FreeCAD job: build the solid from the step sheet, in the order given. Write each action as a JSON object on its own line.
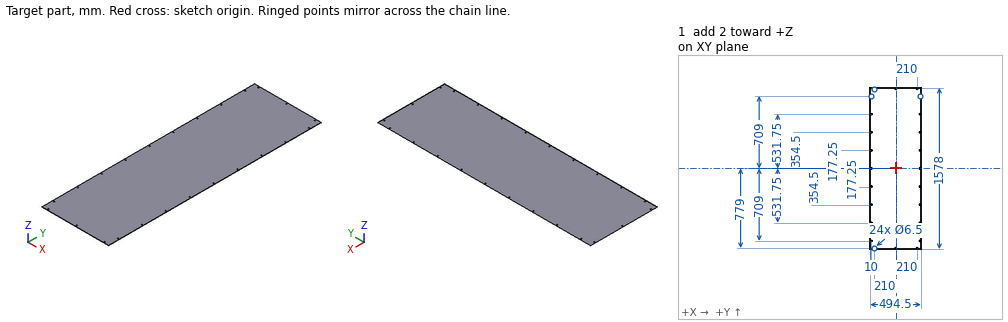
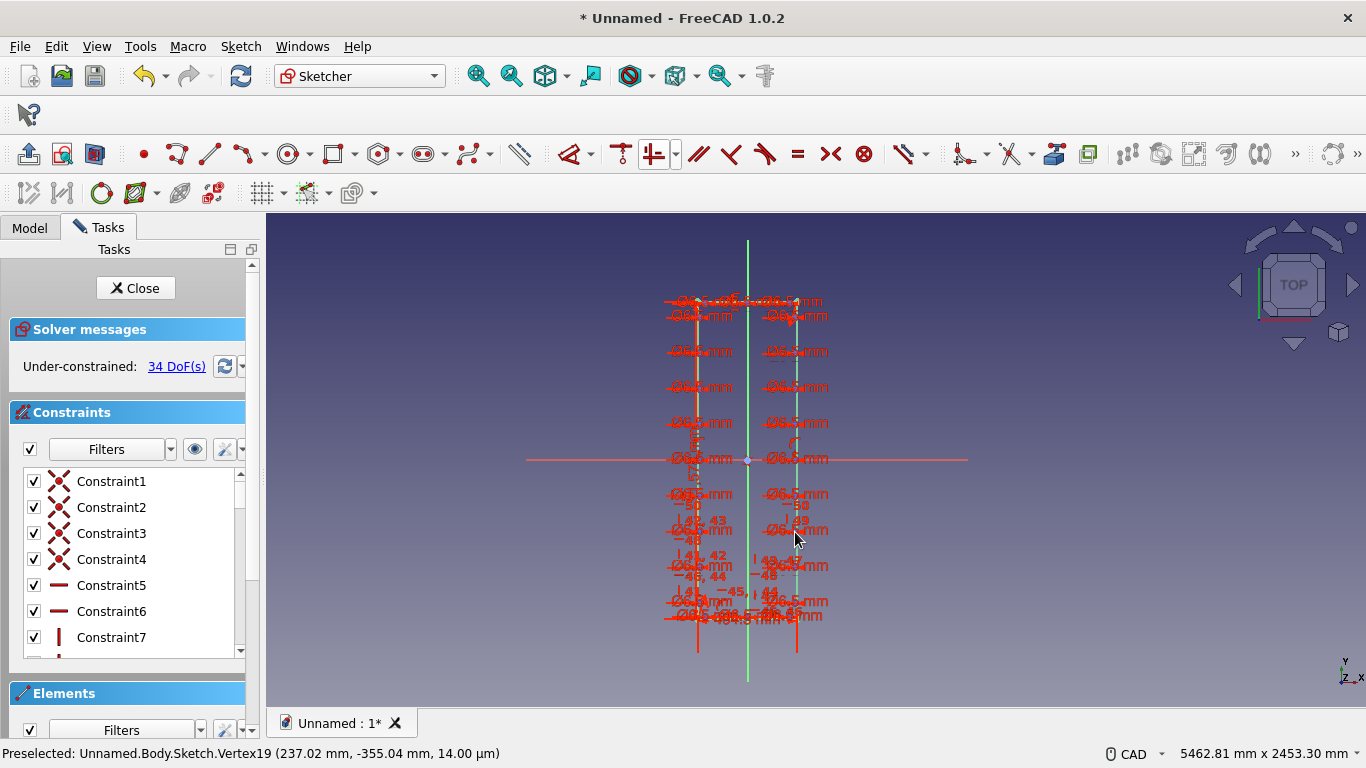
{"action": "left_click", "coordinate": [795, 532]}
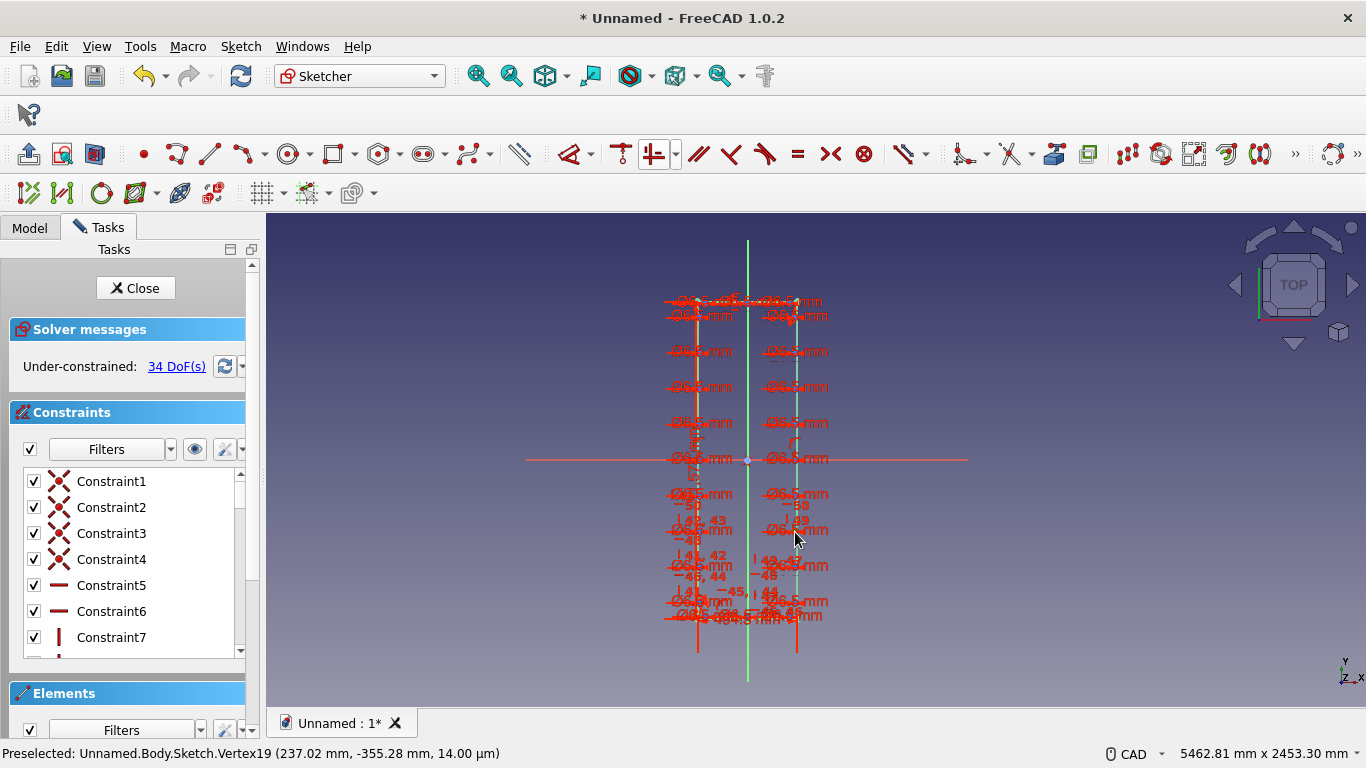
{"action": "left_click", "coordinate": [795, 496]}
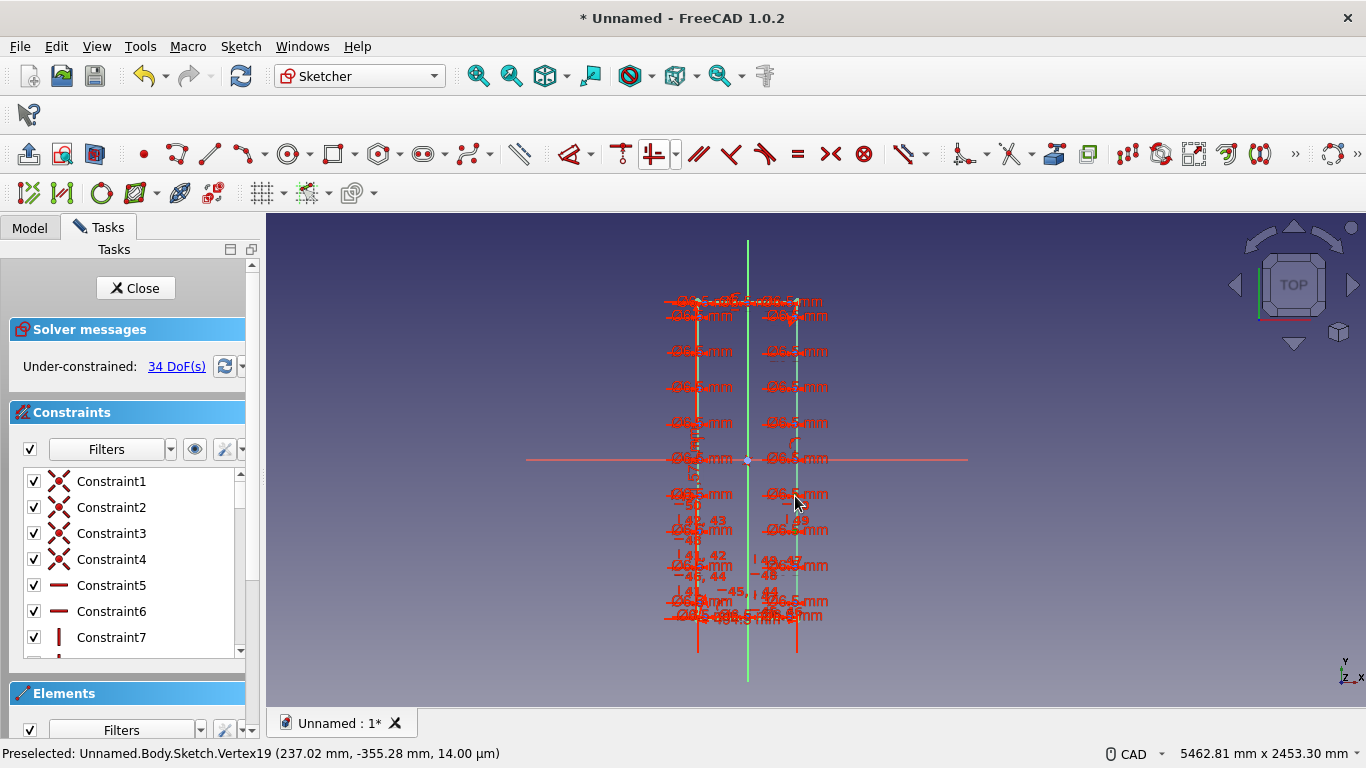
{"action": "key", "text": "v"}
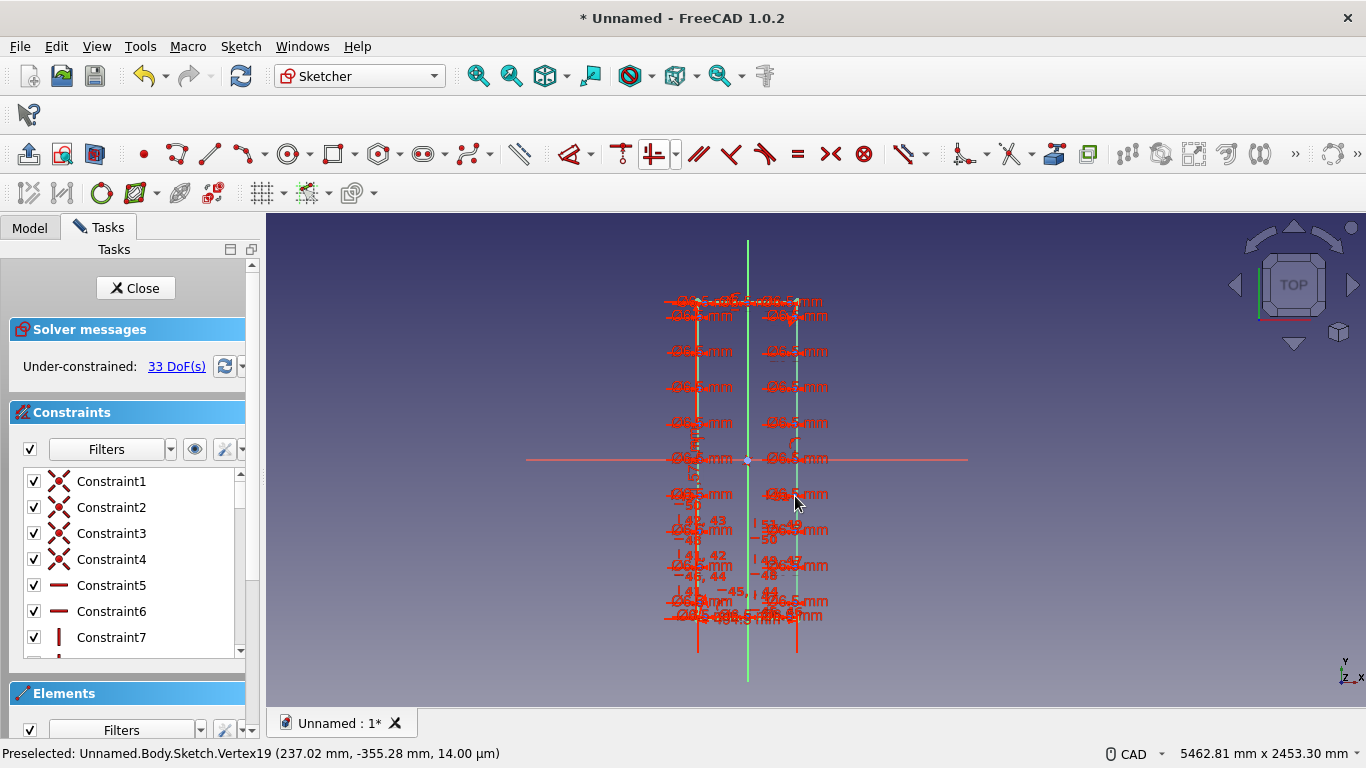
{"action": "left_click", "coordinate": [700, 496]}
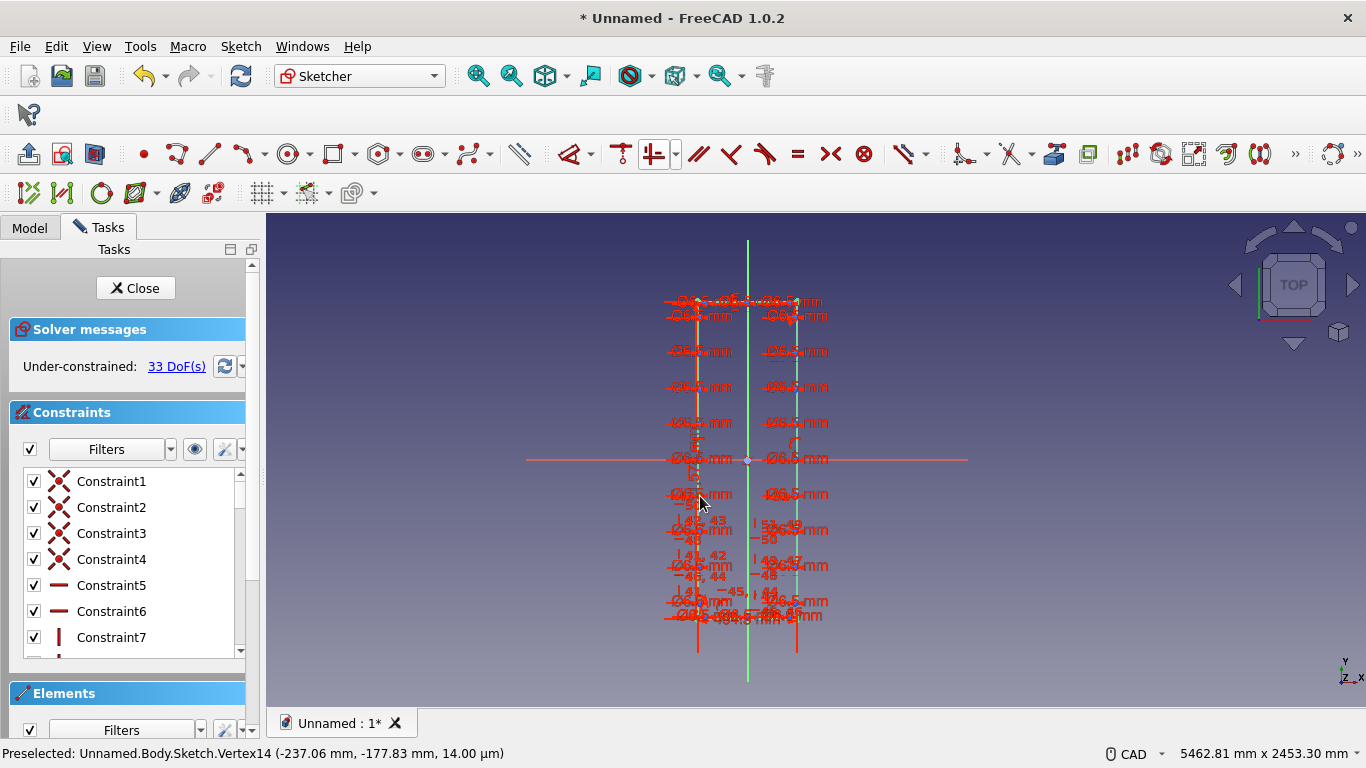
{"action": "left_click", "coordinate": [795, 496]}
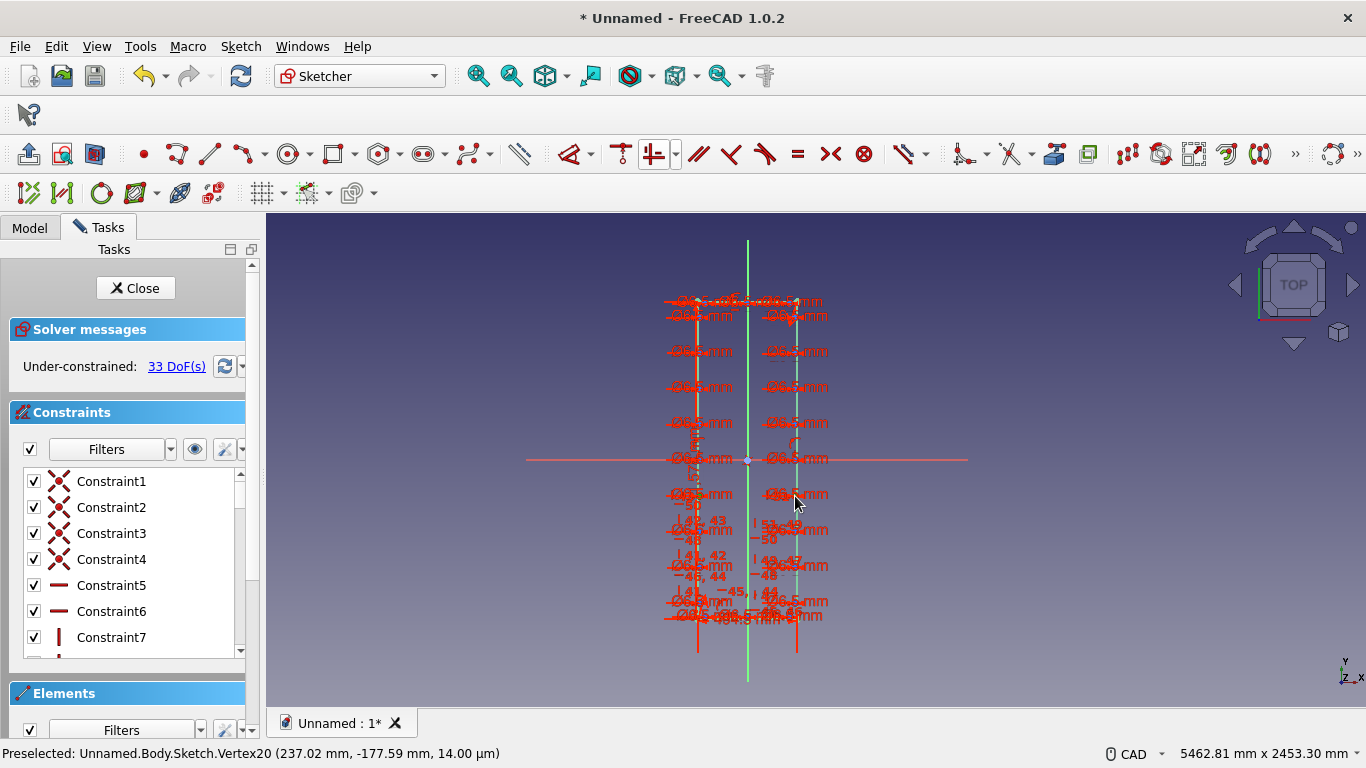
{"action": "key", "text": "h"}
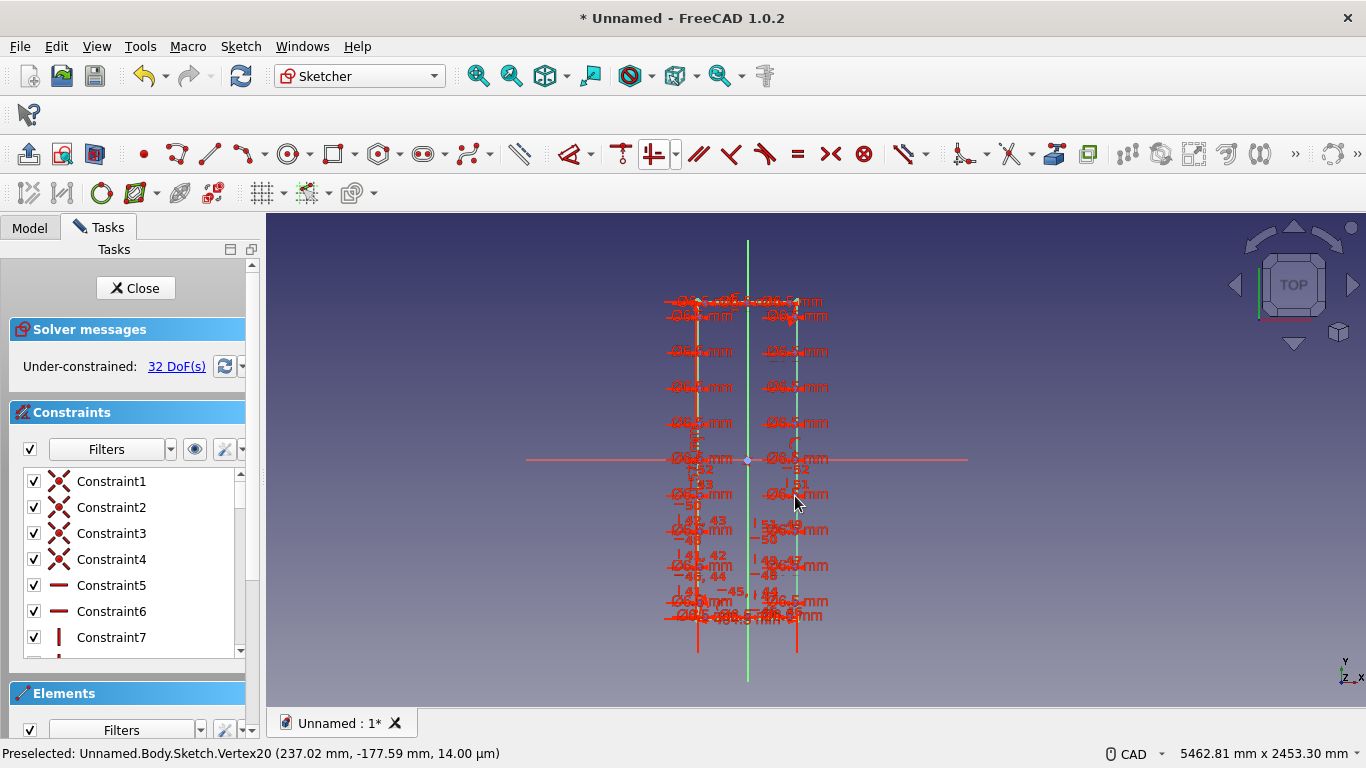
{"action": "left_click", "coordinate": [700, 496]}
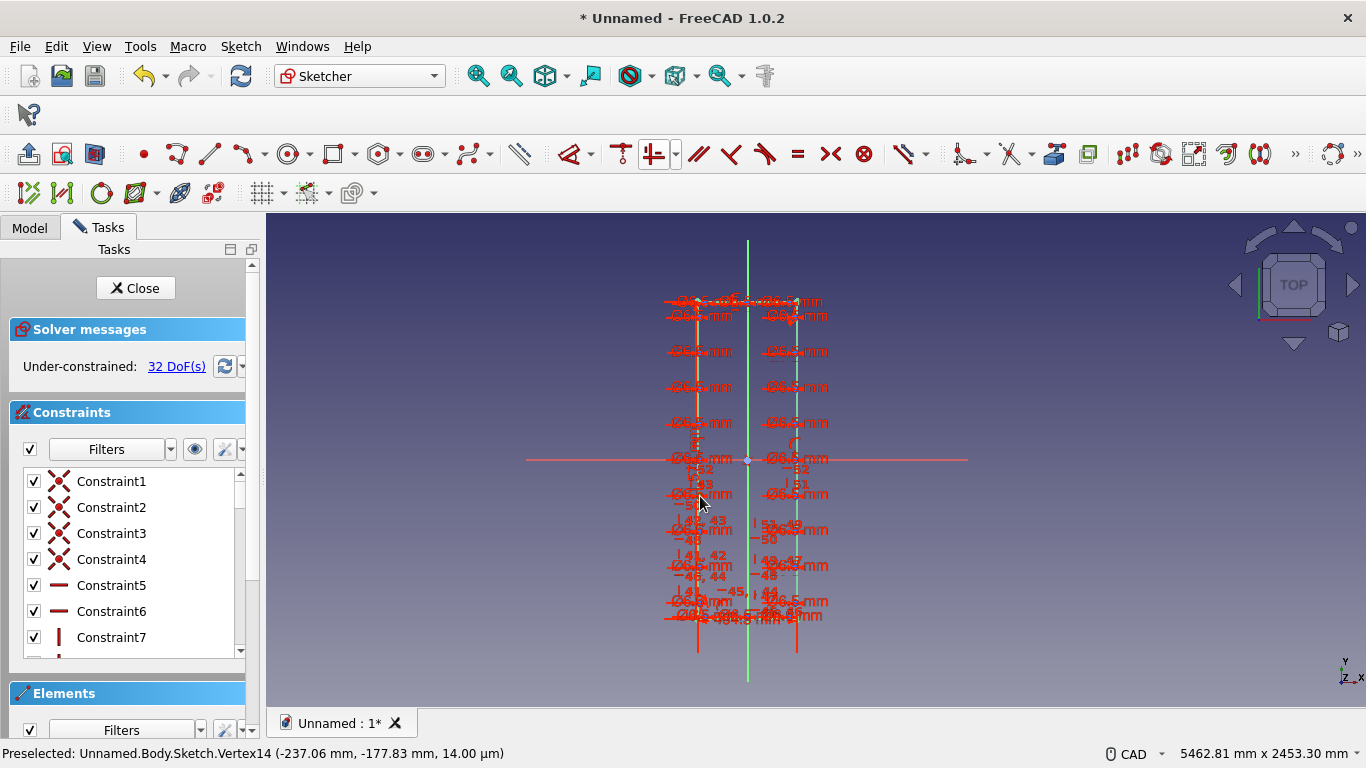
{"action": "left_click", "coordinate": [700, 460]}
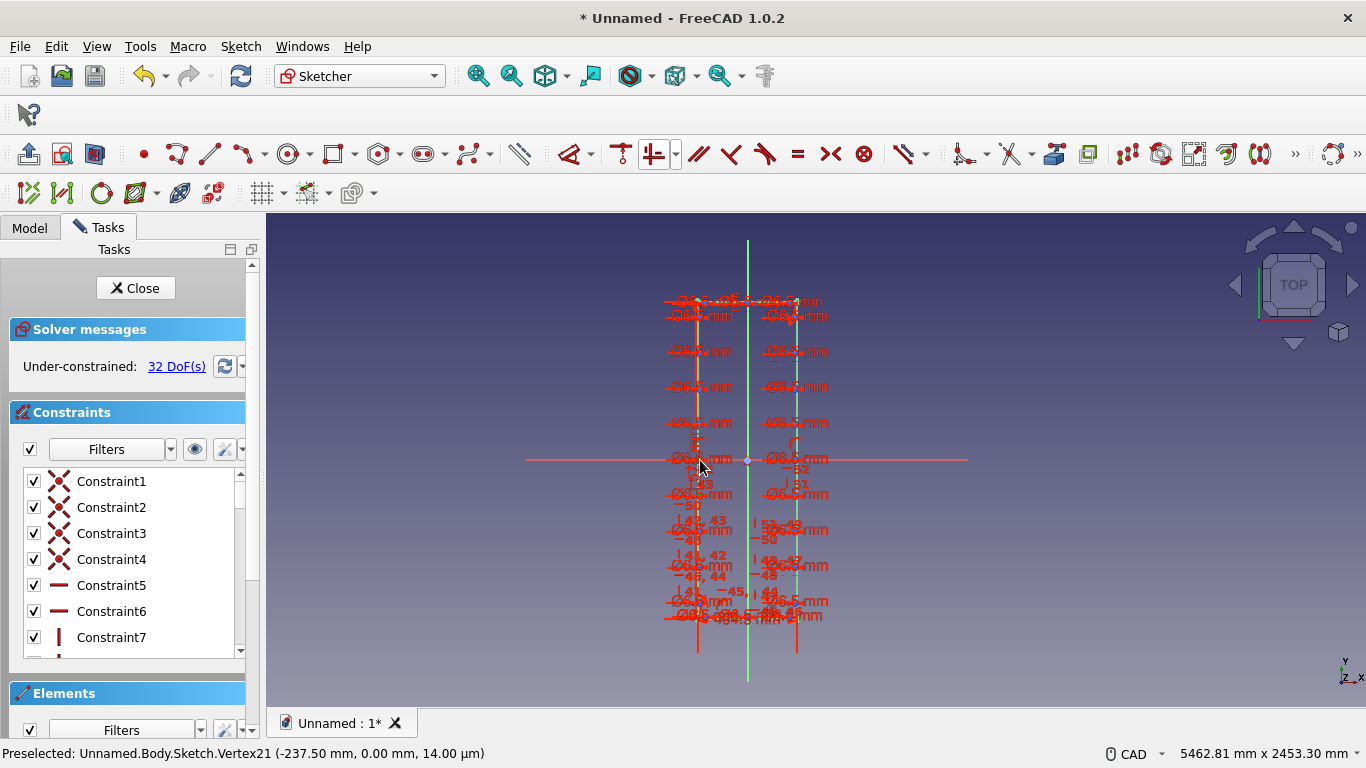
{"action": "key", "text": "v"}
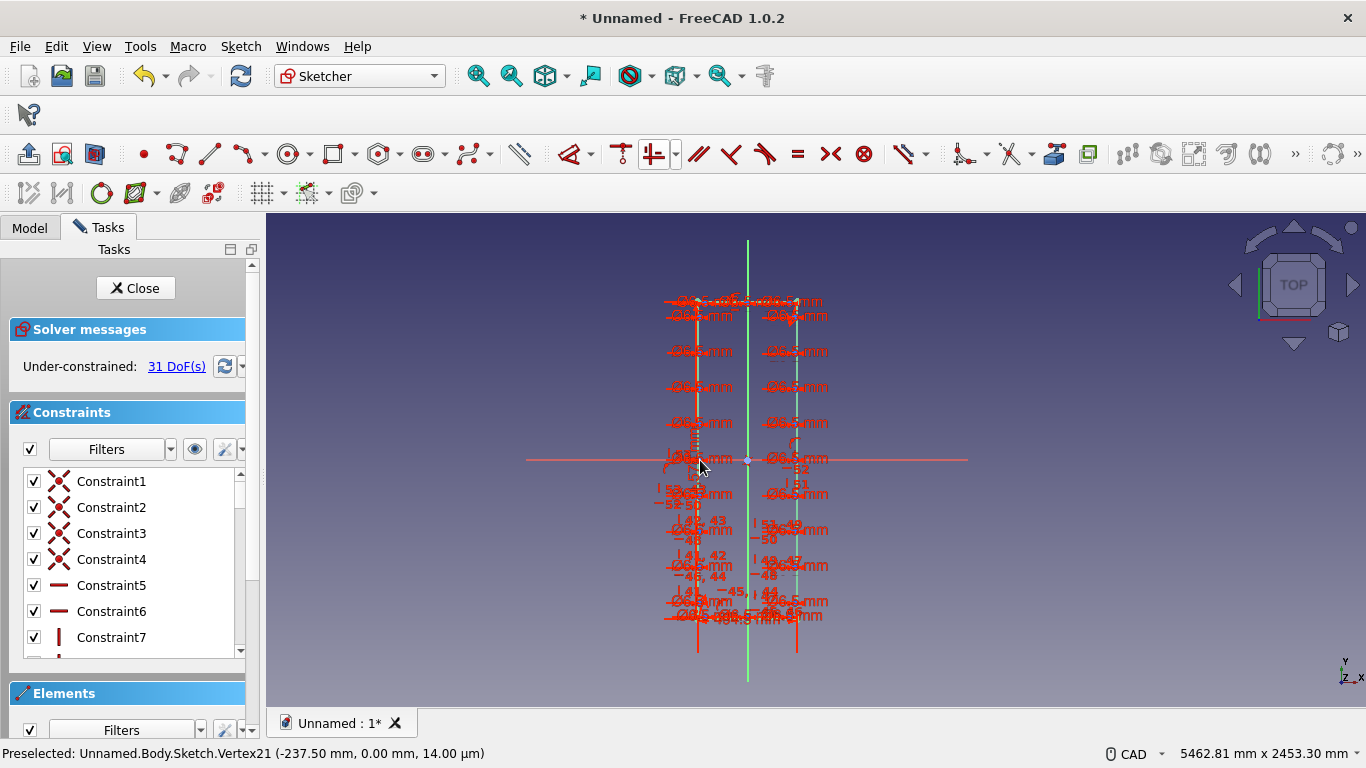
{"action": "left_click", "coordinate": [700, 460]}